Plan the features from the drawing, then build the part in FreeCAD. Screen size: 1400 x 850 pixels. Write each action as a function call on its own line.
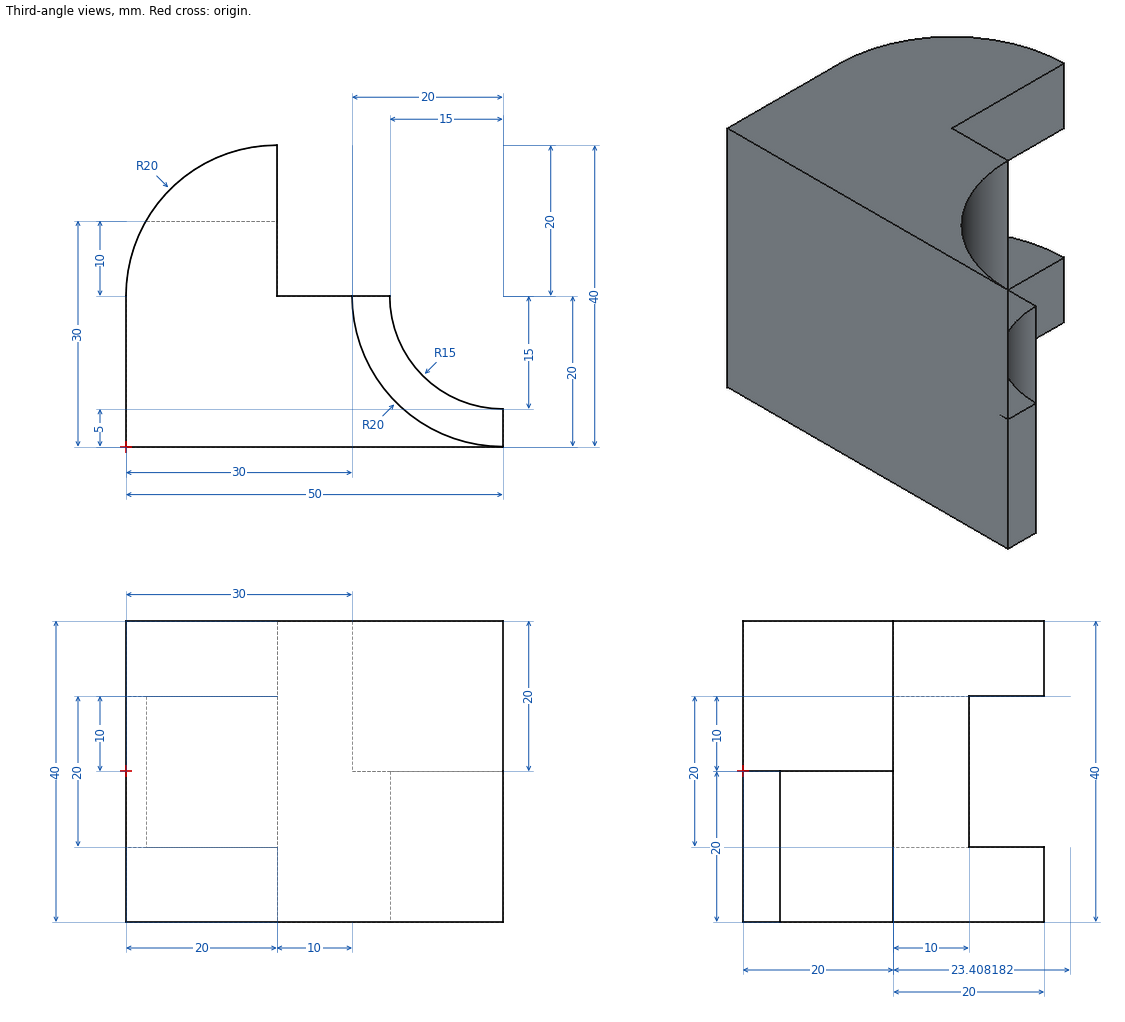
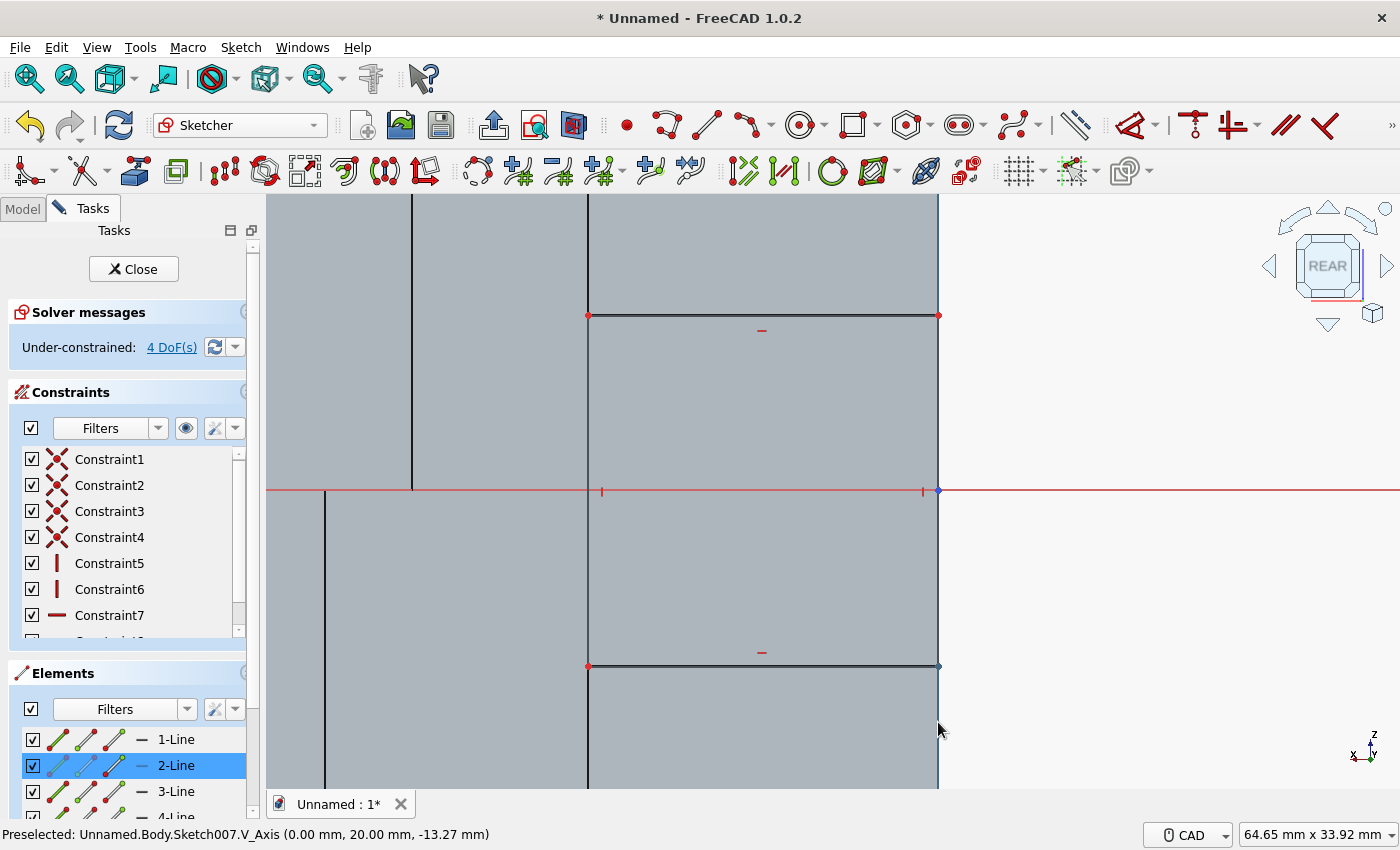
key(c)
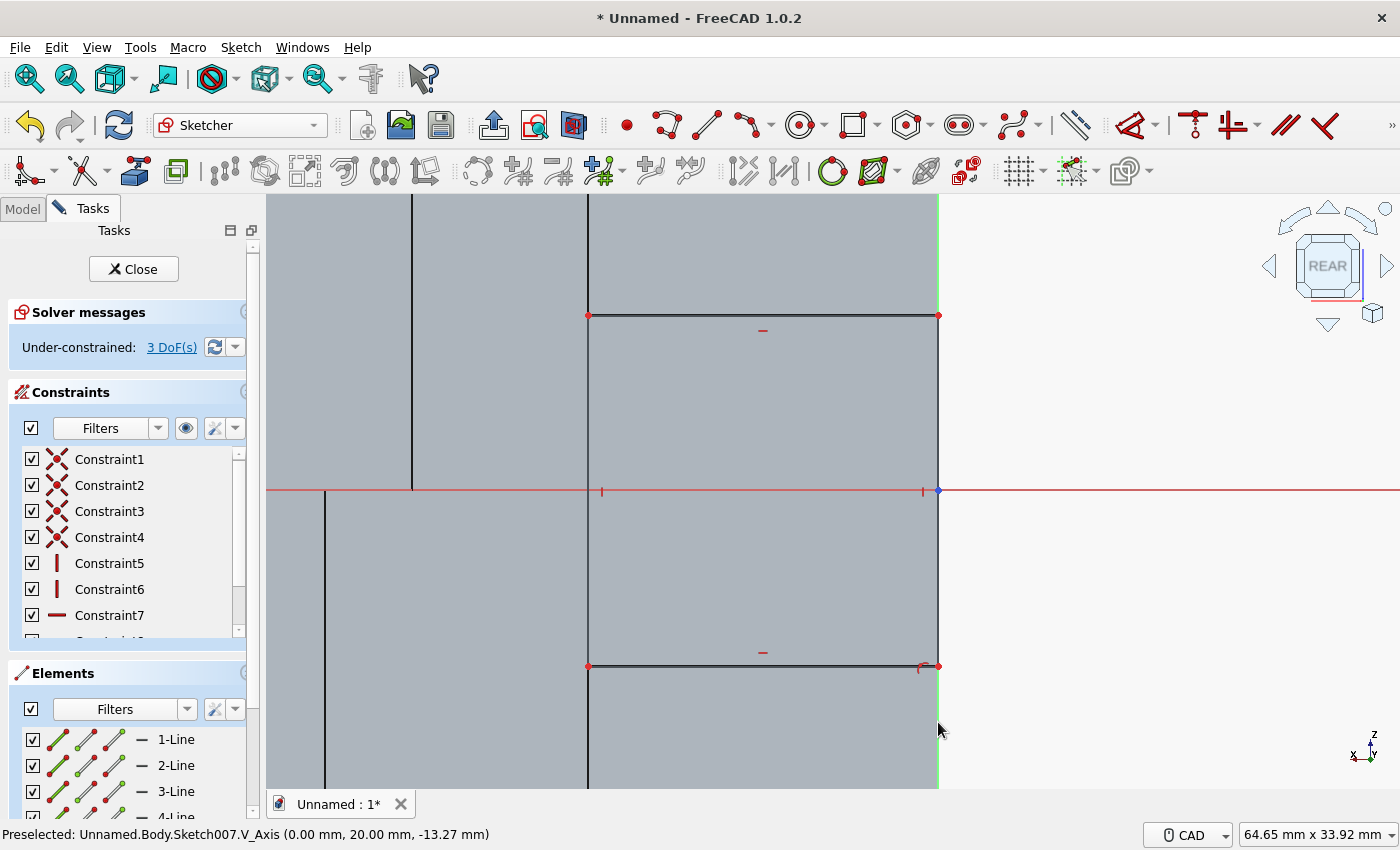
click(1130, 126)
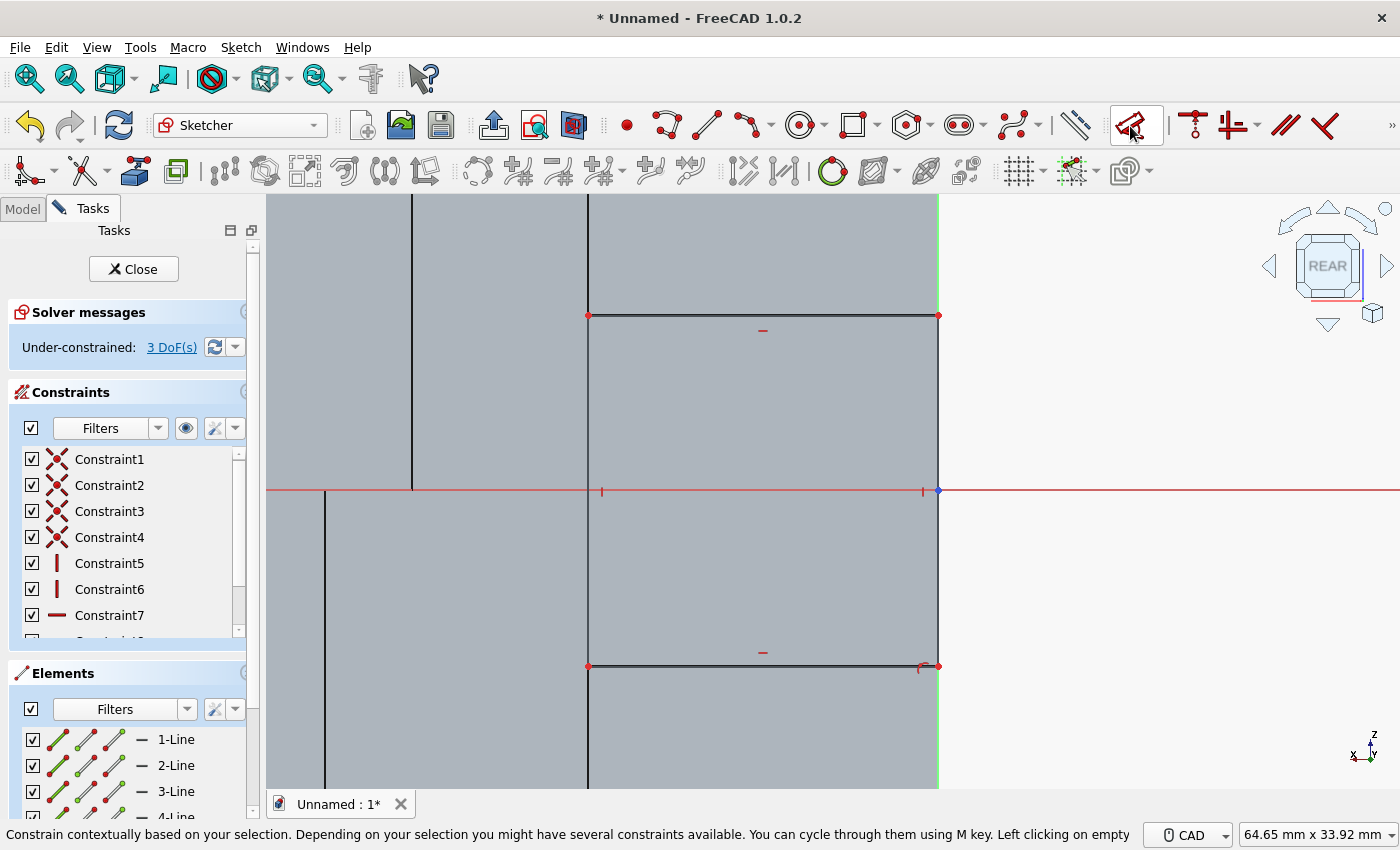
click(588, 421)
click(554, 411)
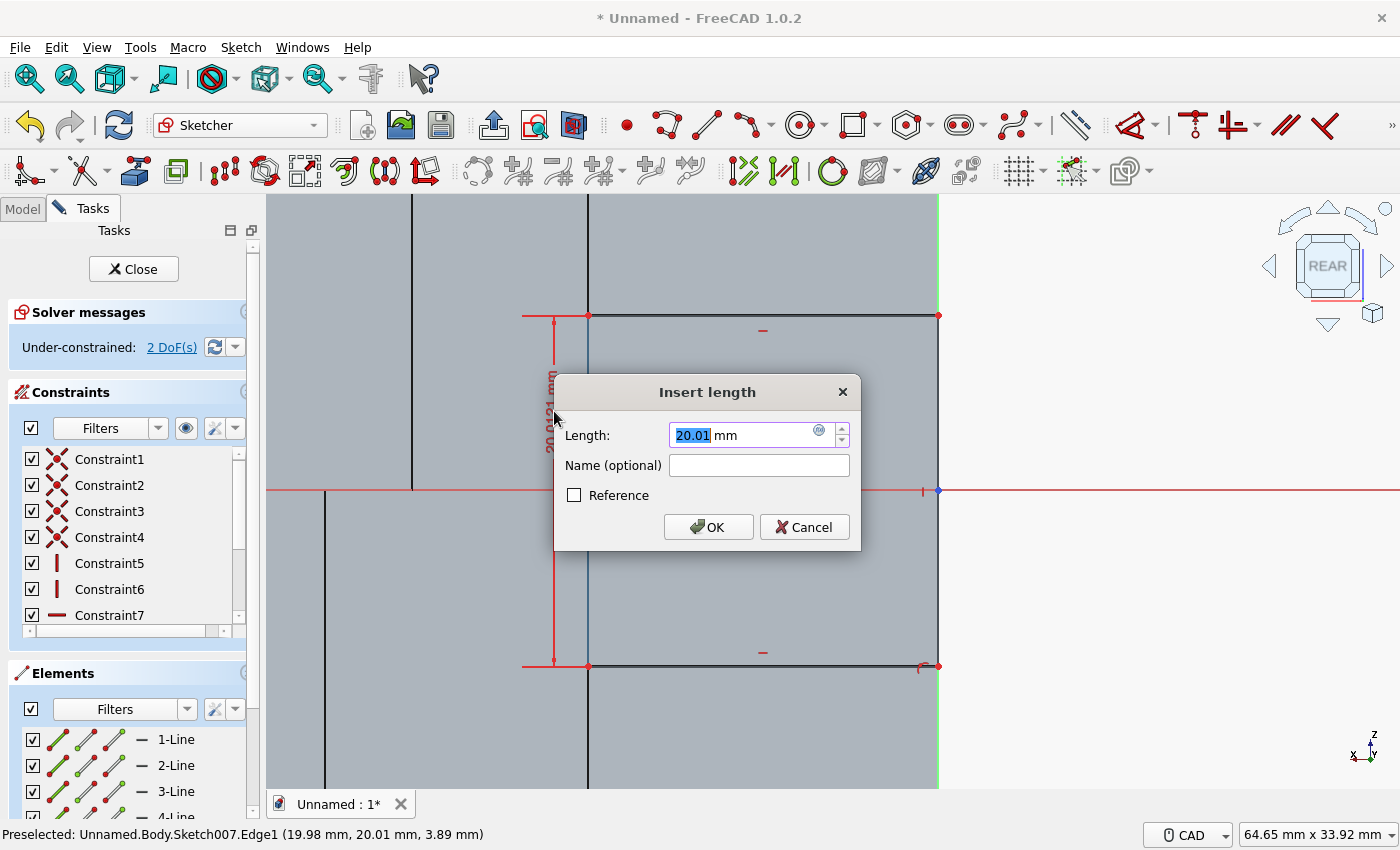
text(20)
key(Return)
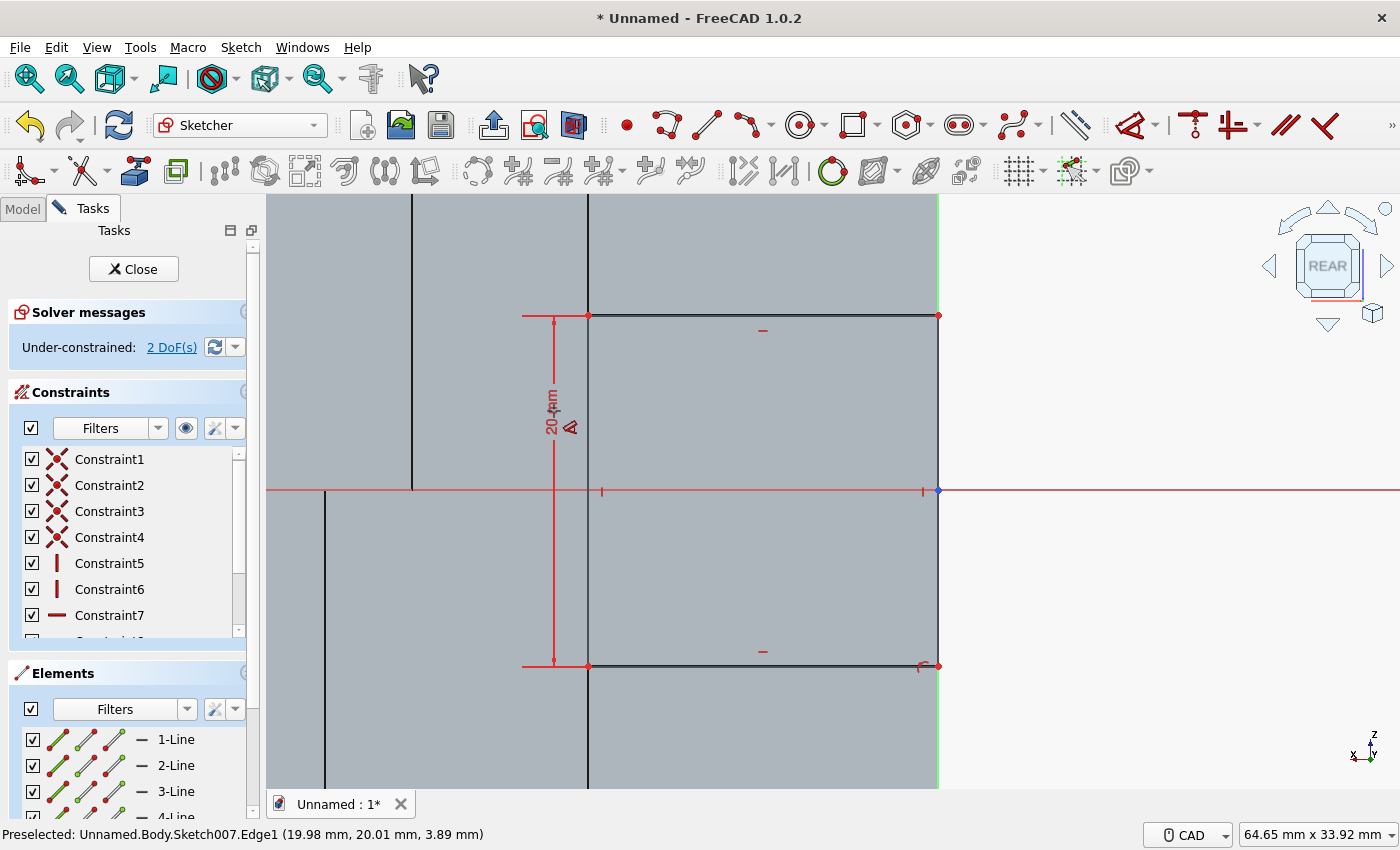
click(693, 667)
click(763, 701)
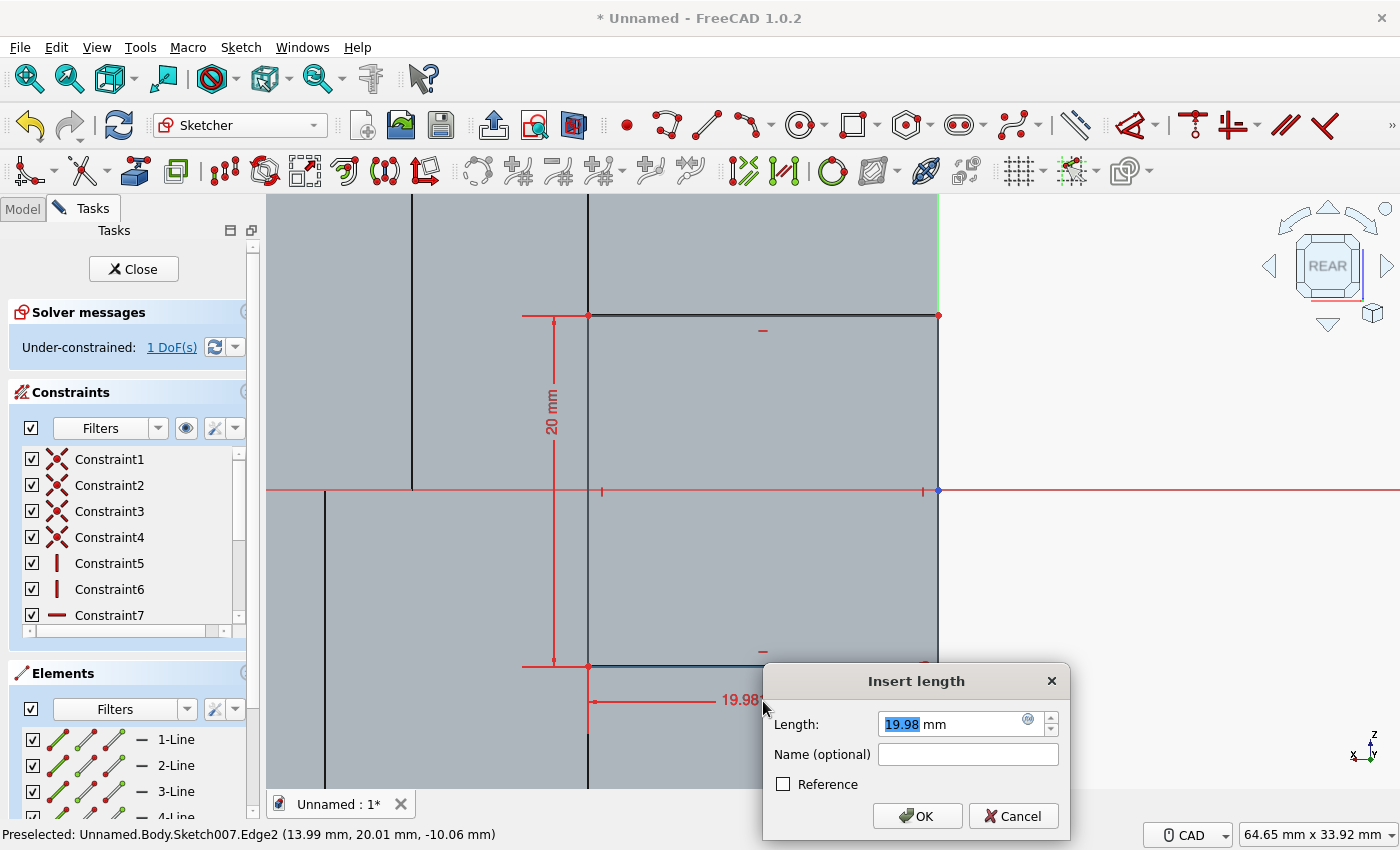
text(20)
key(Return)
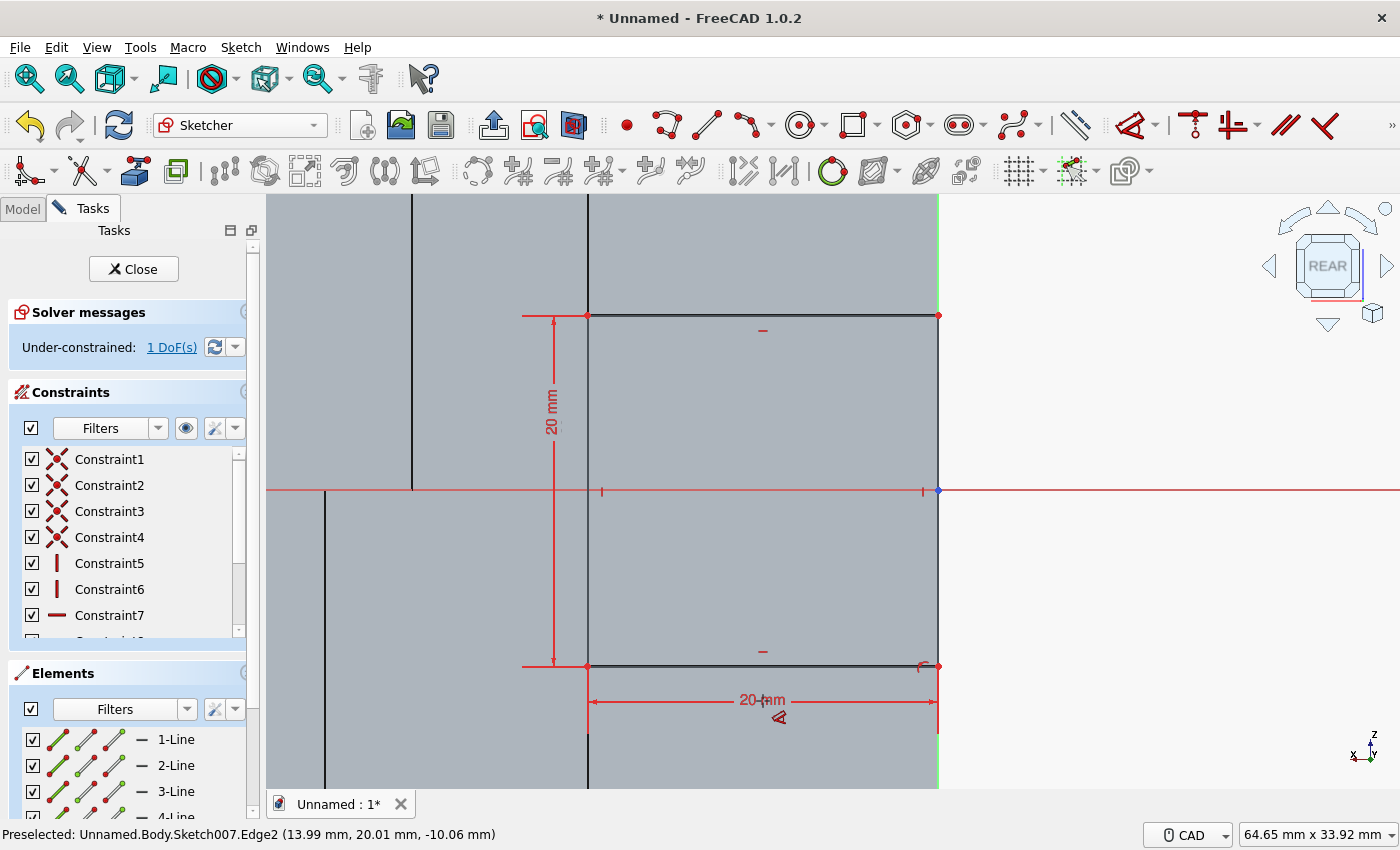
click(588, 316)
click(972, 403)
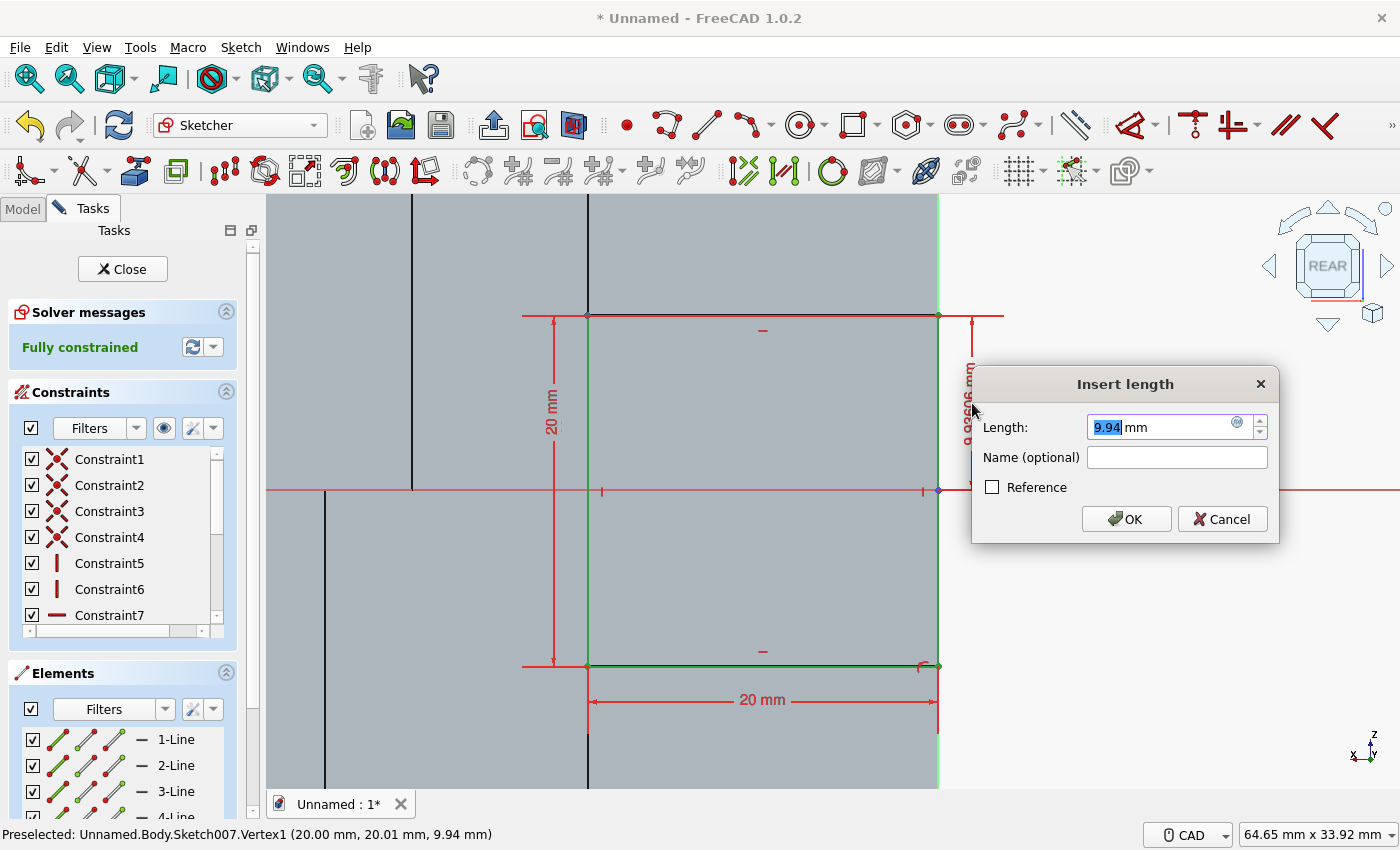
text(10)
key(Return)
key(Escape)